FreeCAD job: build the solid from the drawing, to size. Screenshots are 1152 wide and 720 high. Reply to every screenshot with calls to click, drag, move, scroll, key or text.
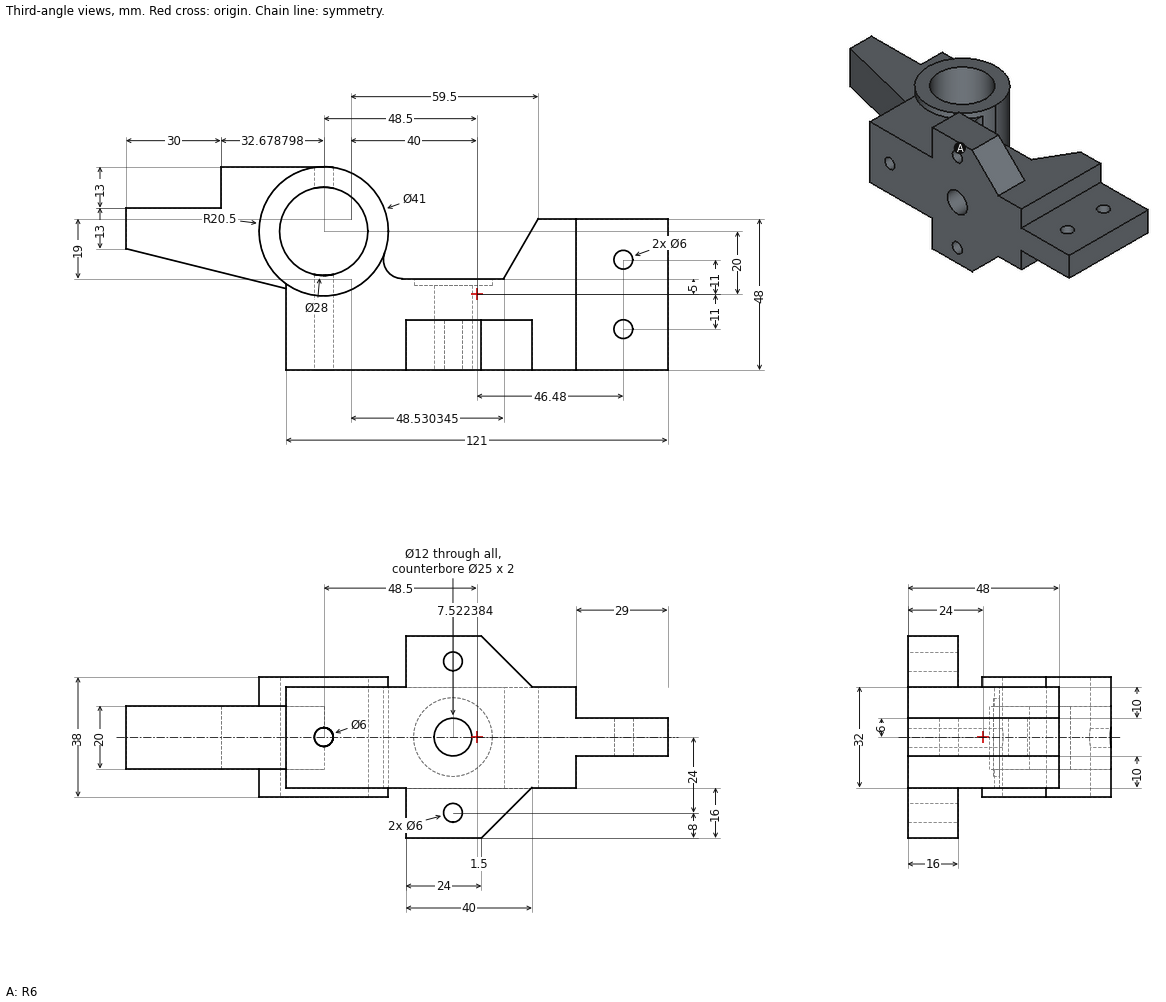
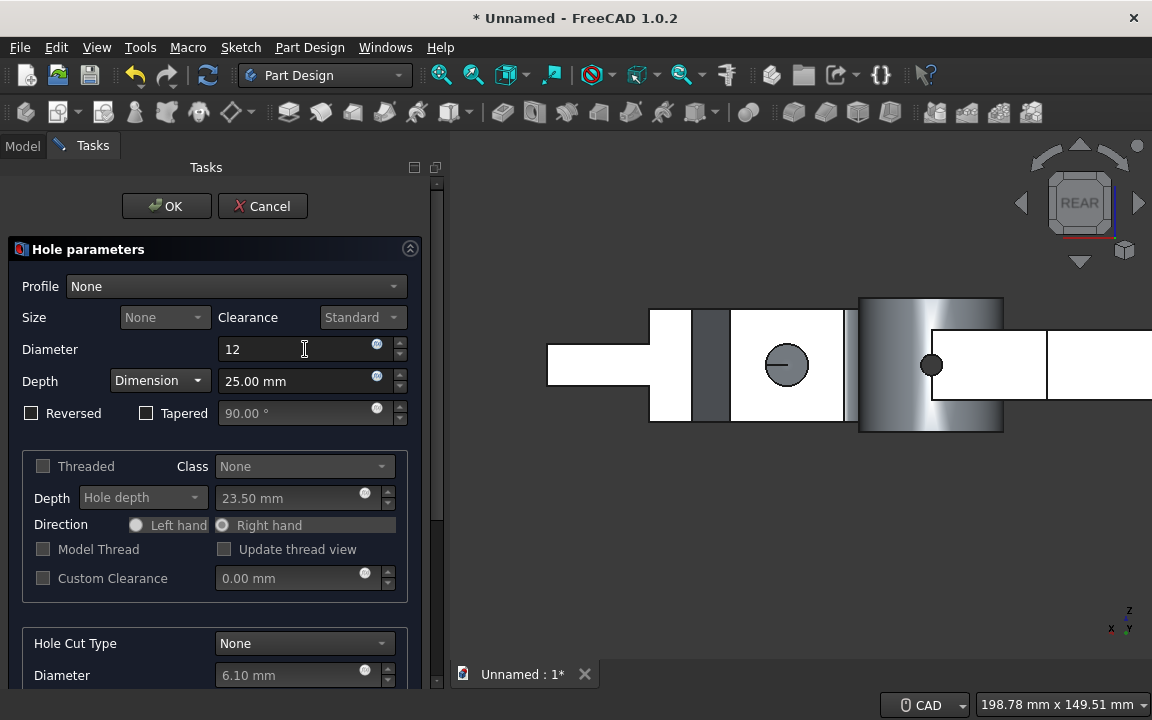
click(161, 380)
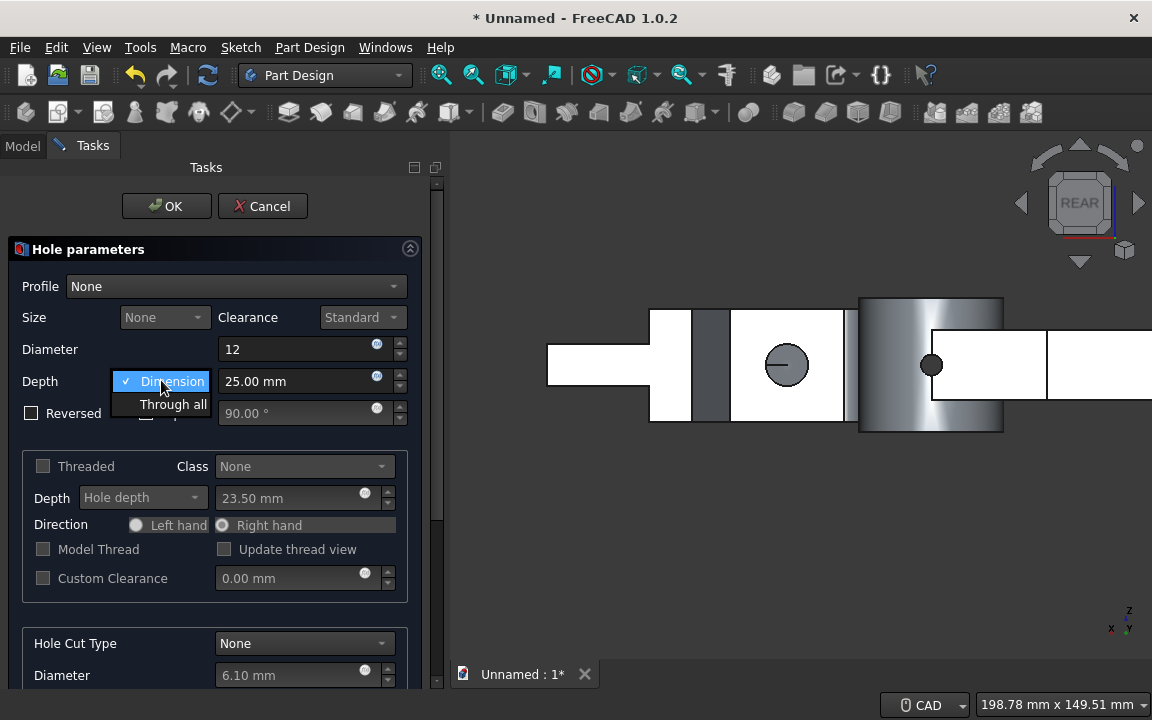
click(160, 404)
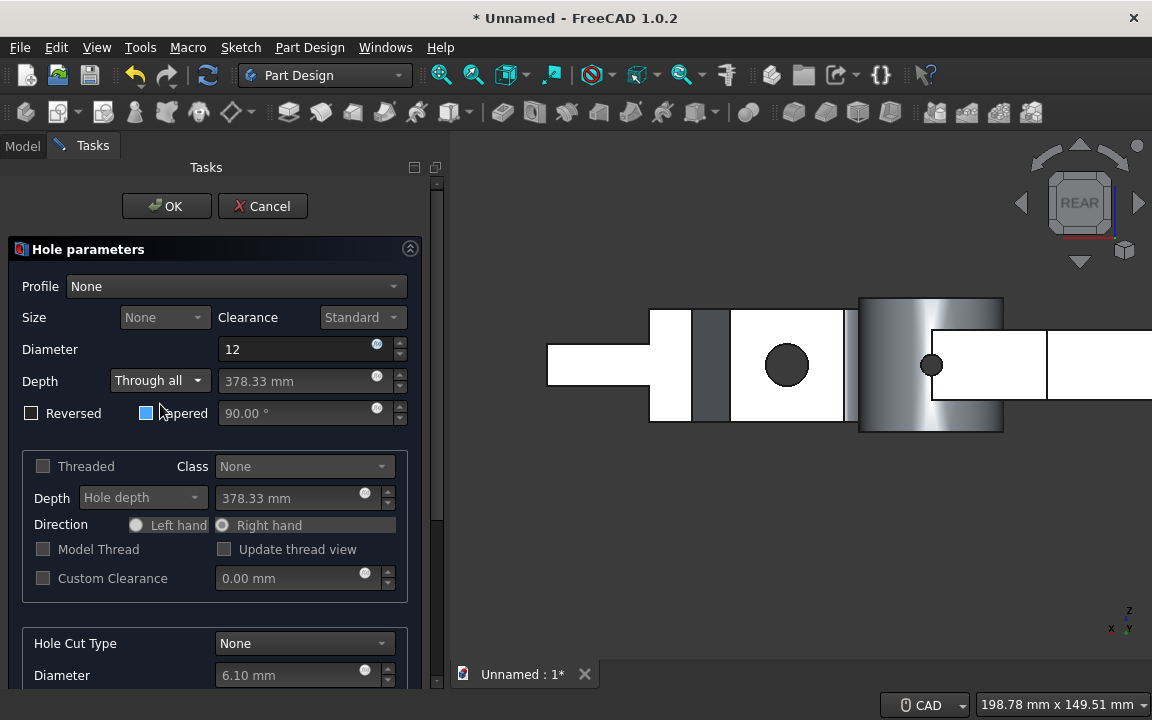
click(306, 644)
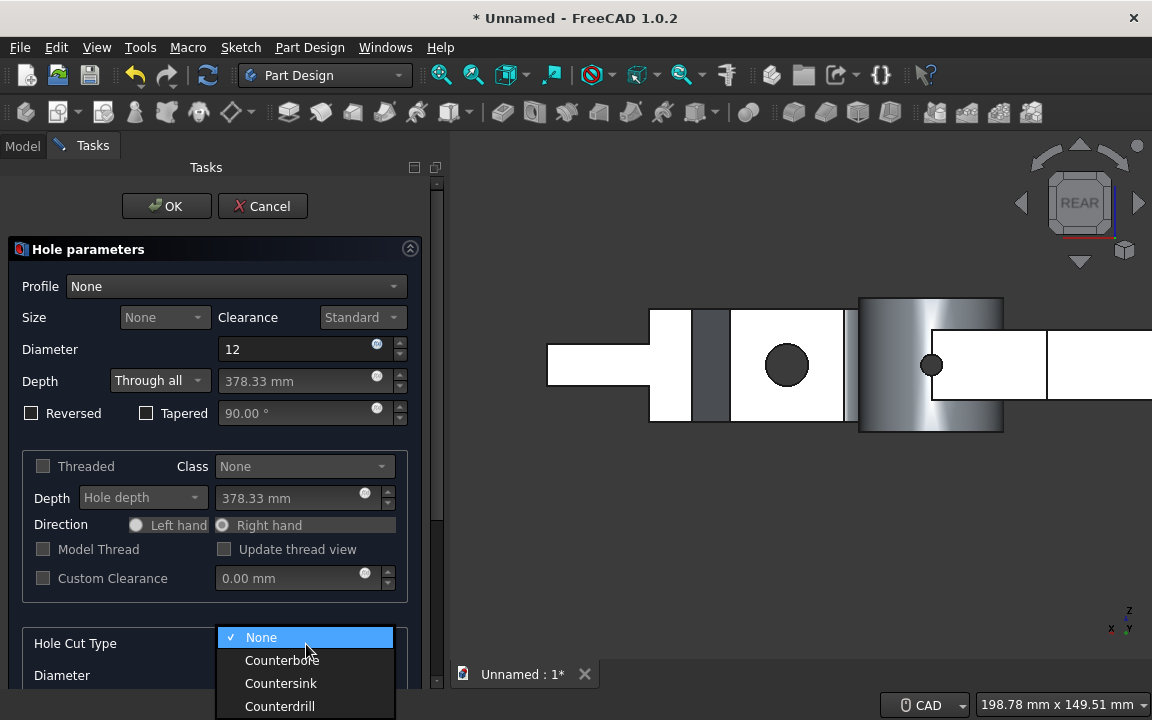
click(304, 660)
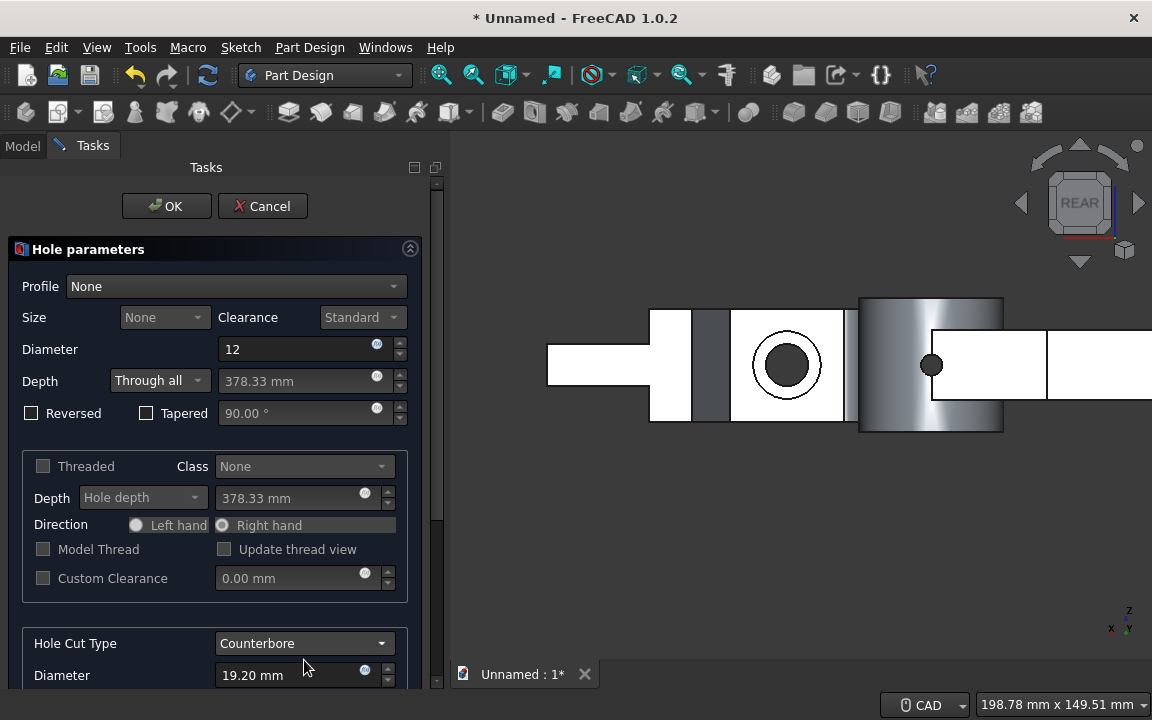
triple_click(298, 675)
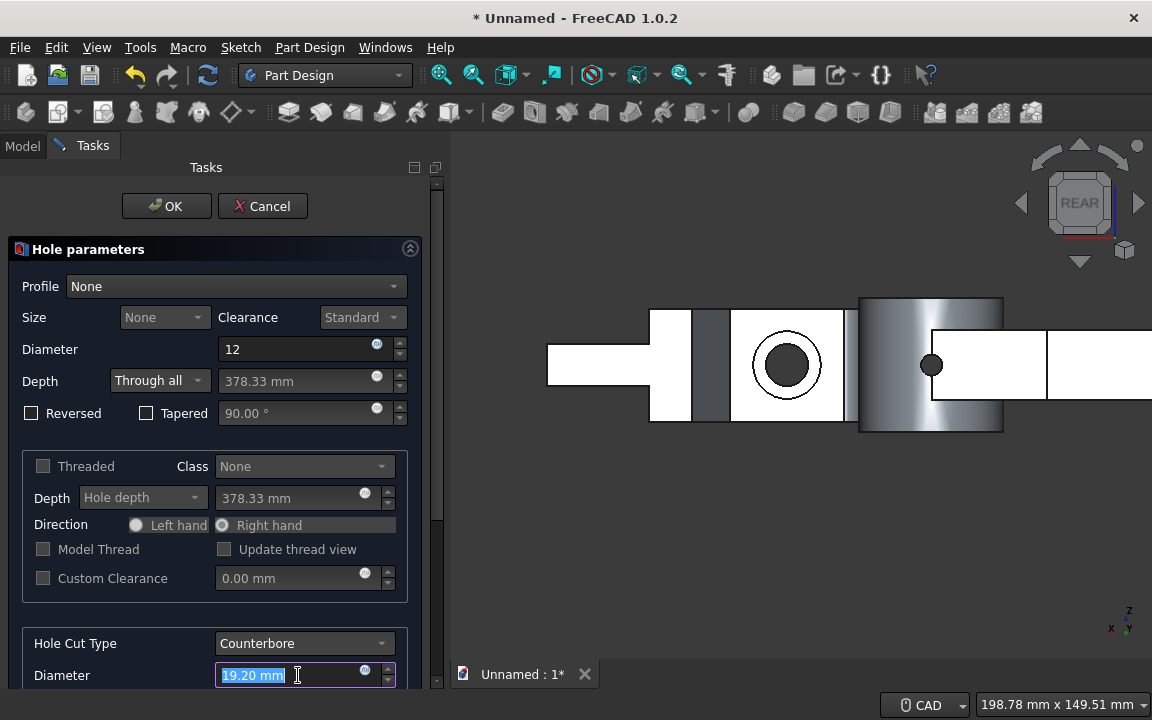
text(25)
key(Tab)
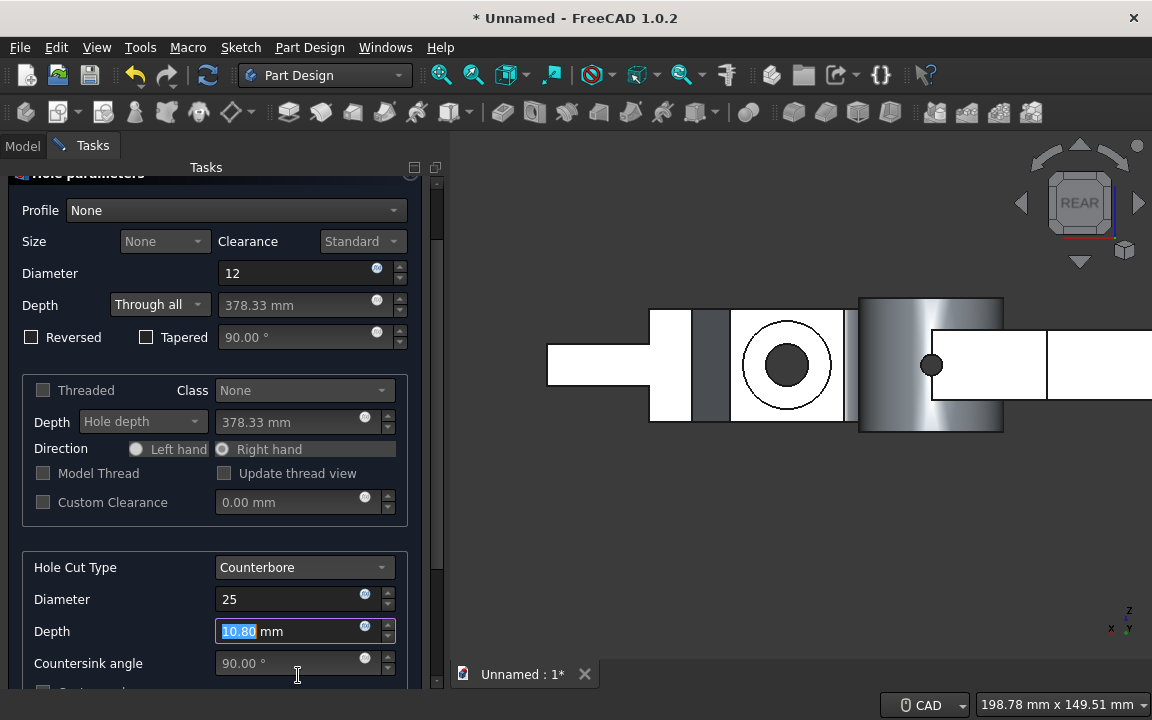
text(2)
key(Tab)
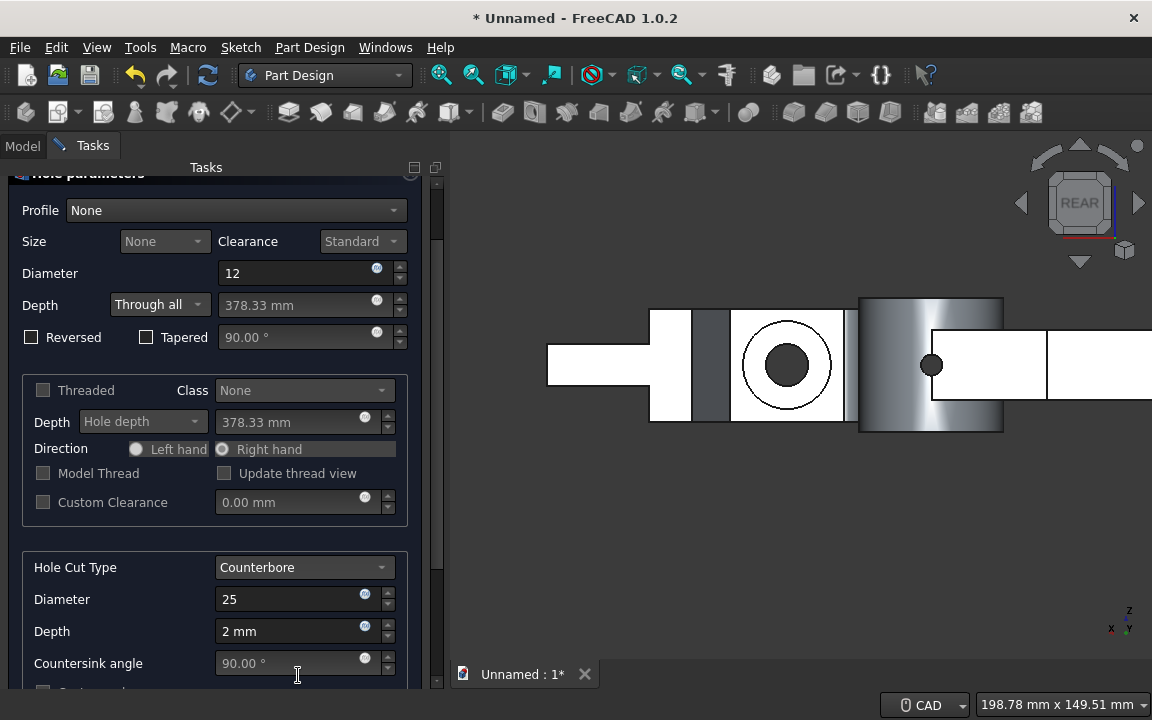
scroll(437, 432, up, 3)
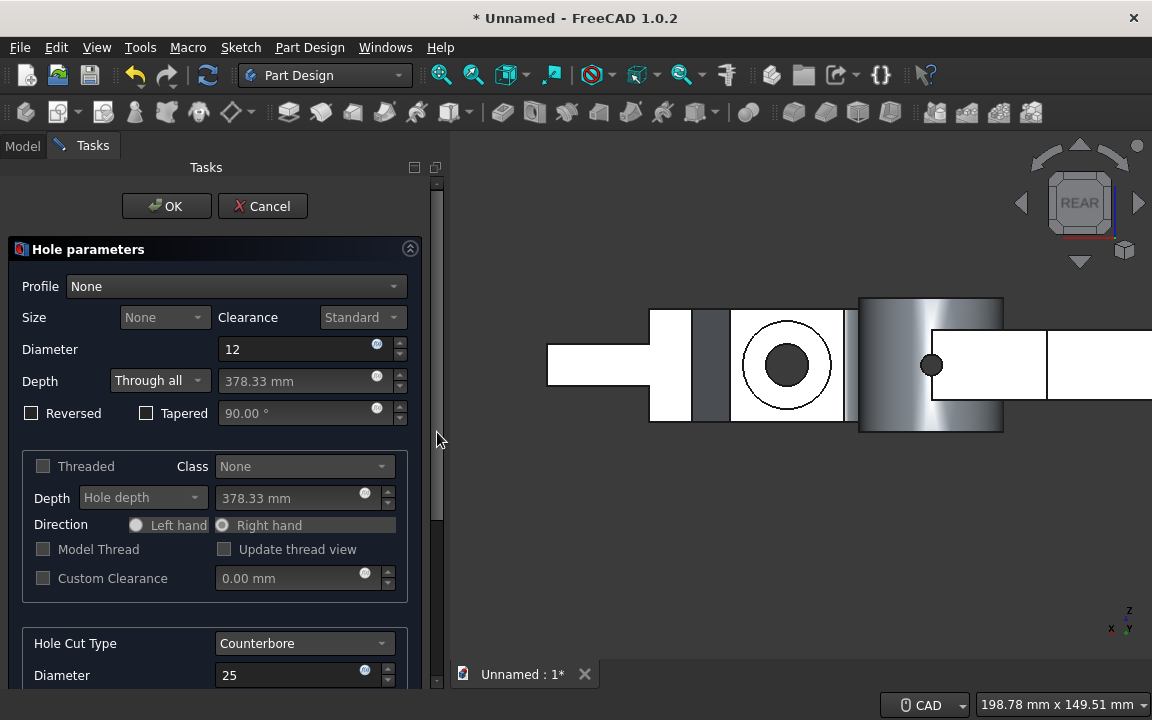
click(167, 206)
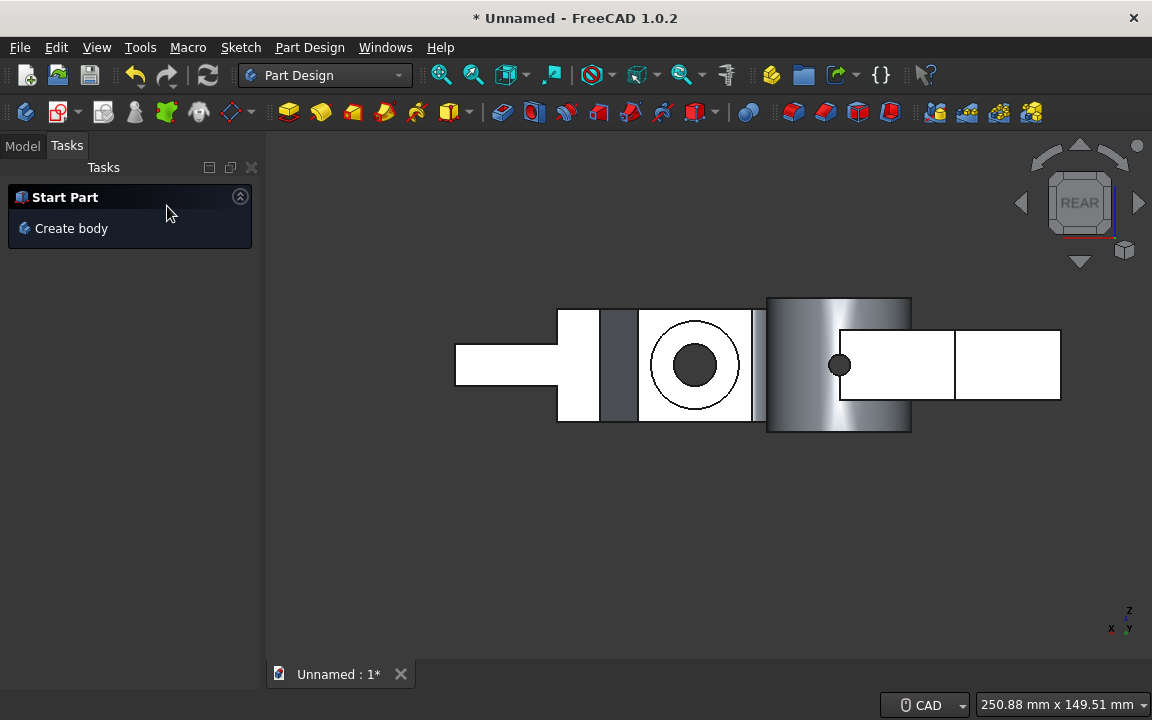
key(0)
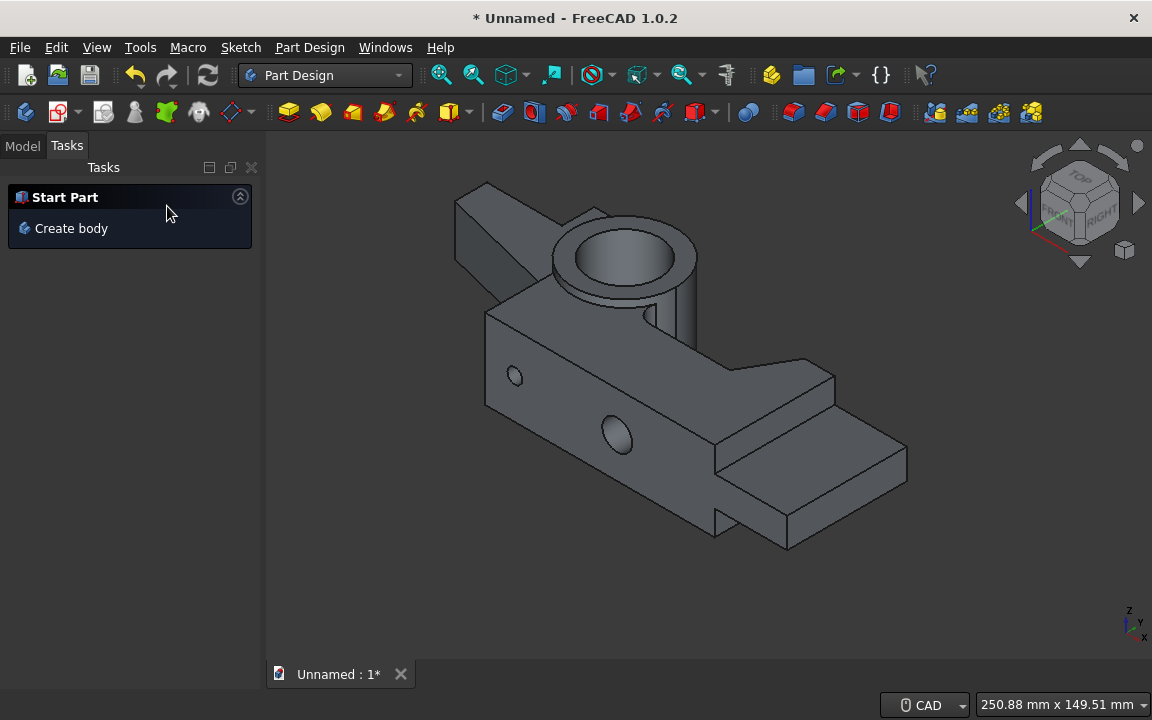
click(679, 470)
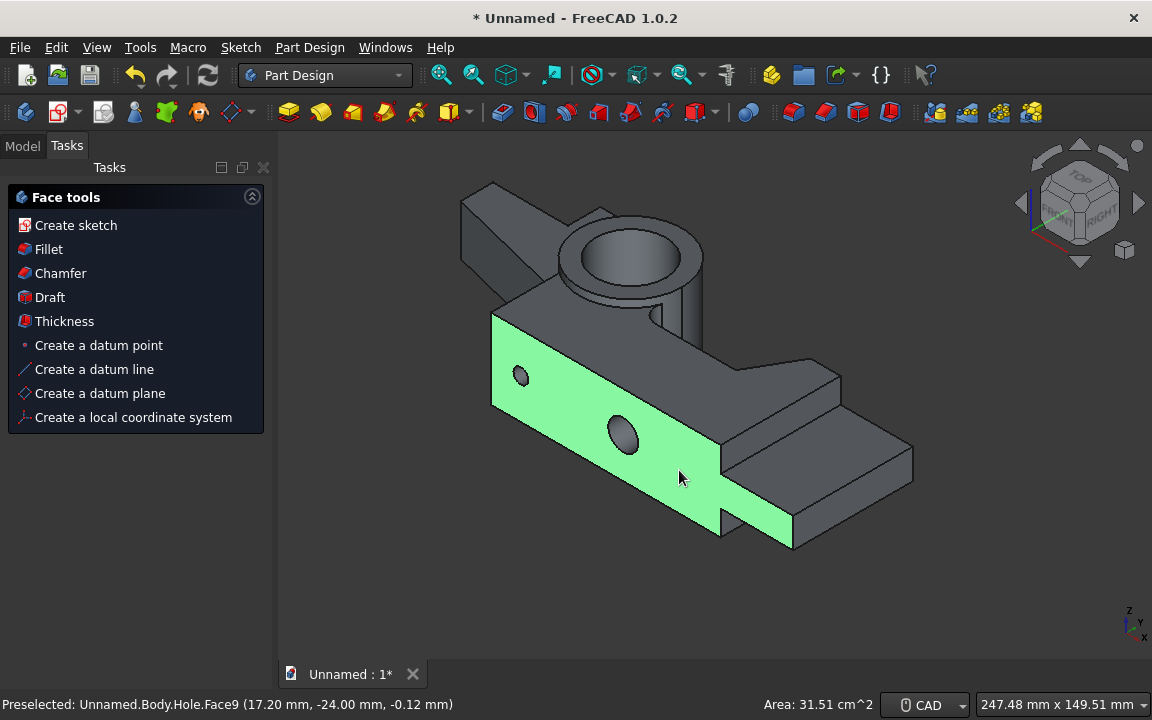
click(58, 112)